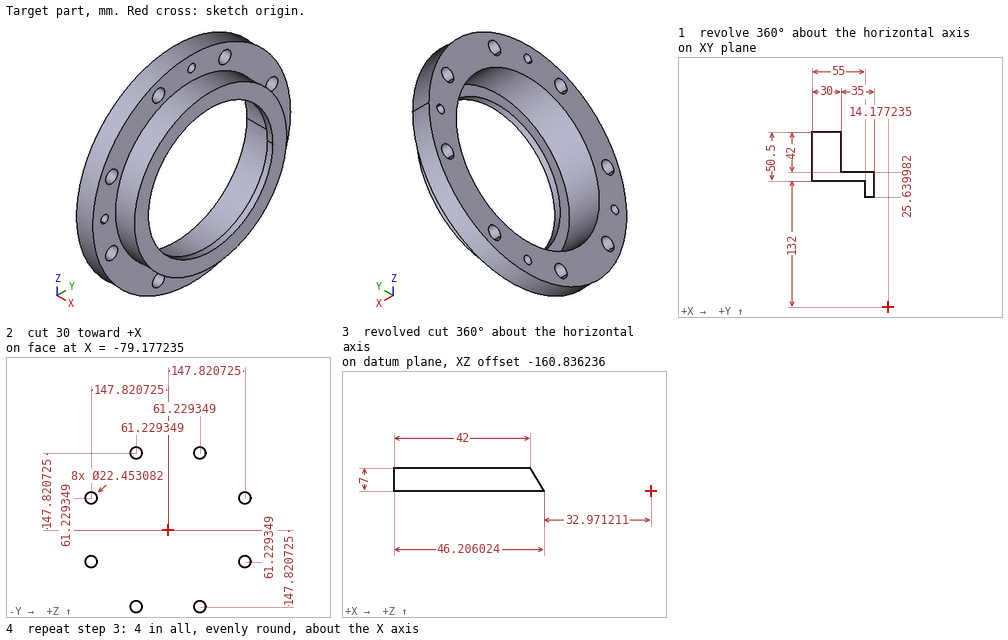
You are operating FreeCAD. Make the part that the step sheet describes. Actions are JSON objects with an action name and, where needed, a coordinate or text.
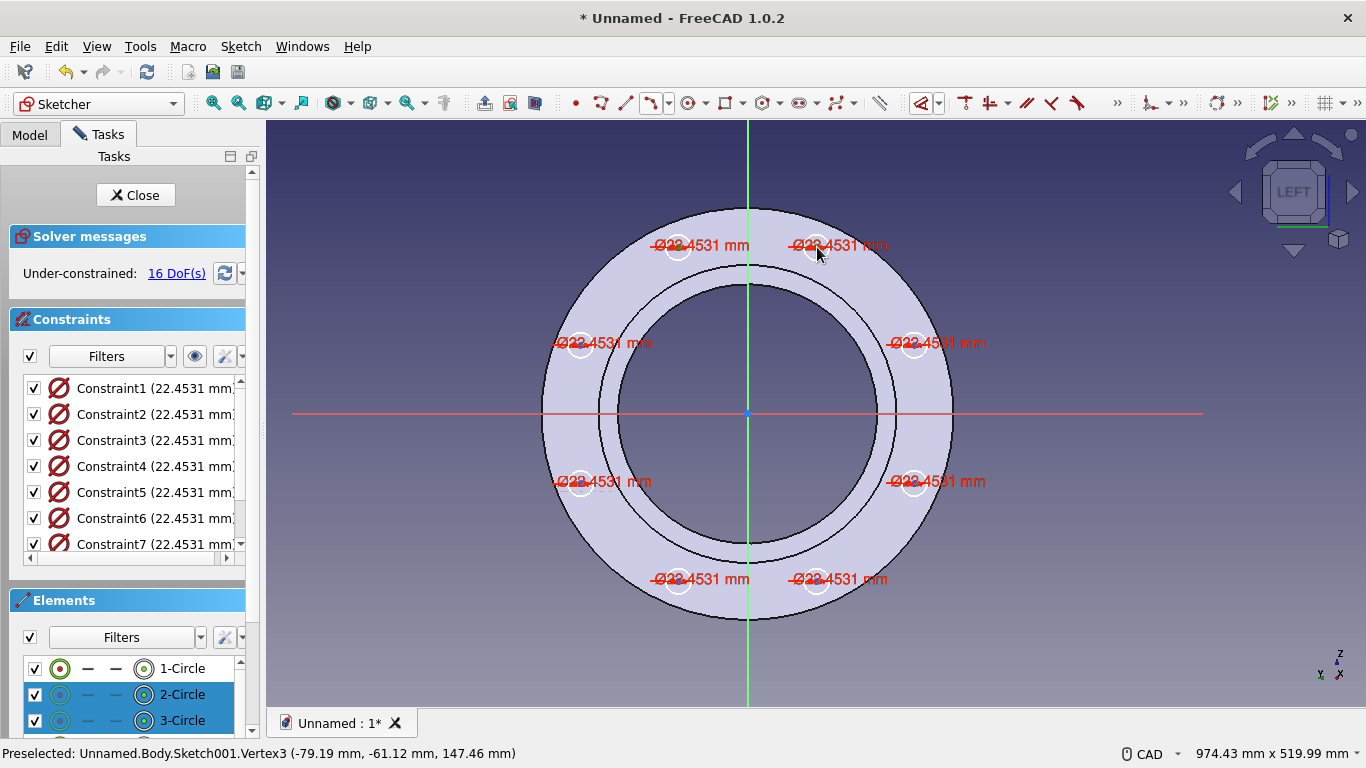
{"action": "left_click", "coordinate": [1008, 104]}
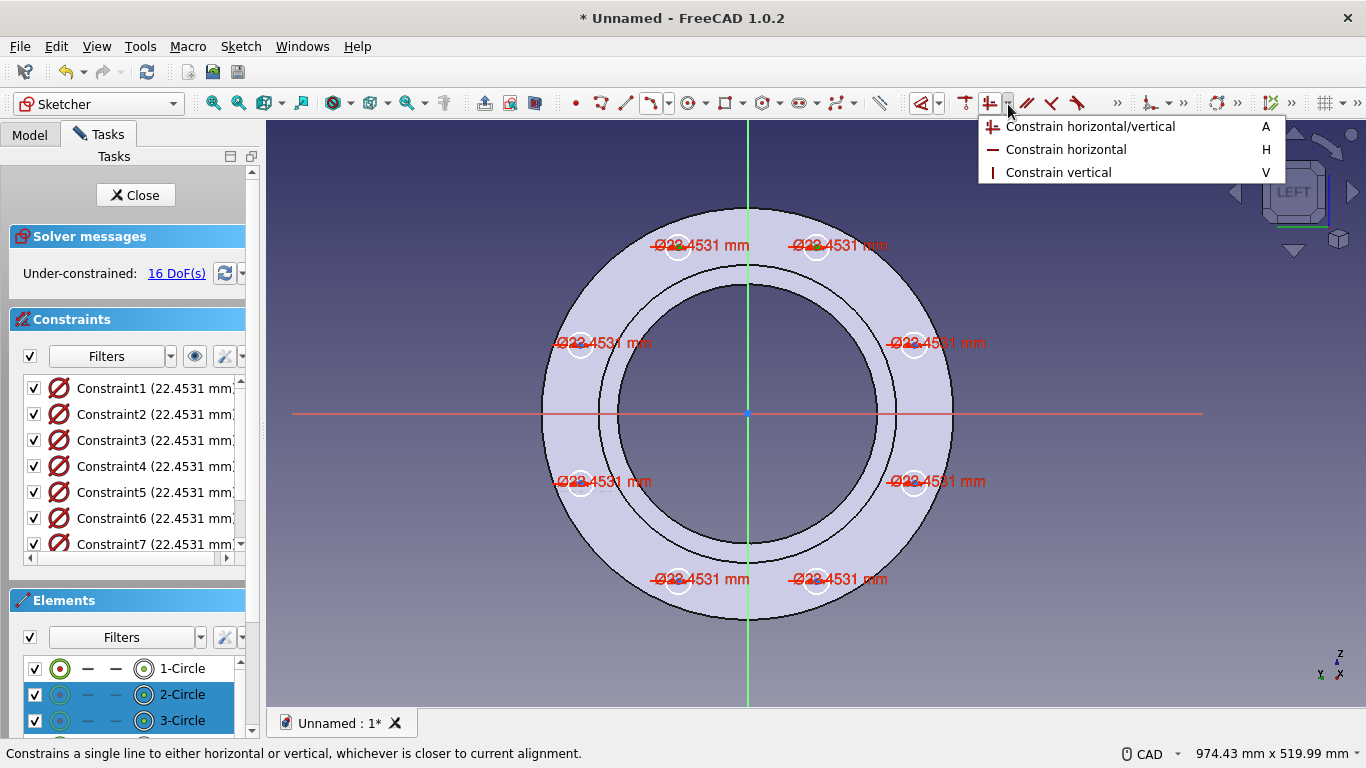
{"action": "left_click", "coordinate": [1132, 150]}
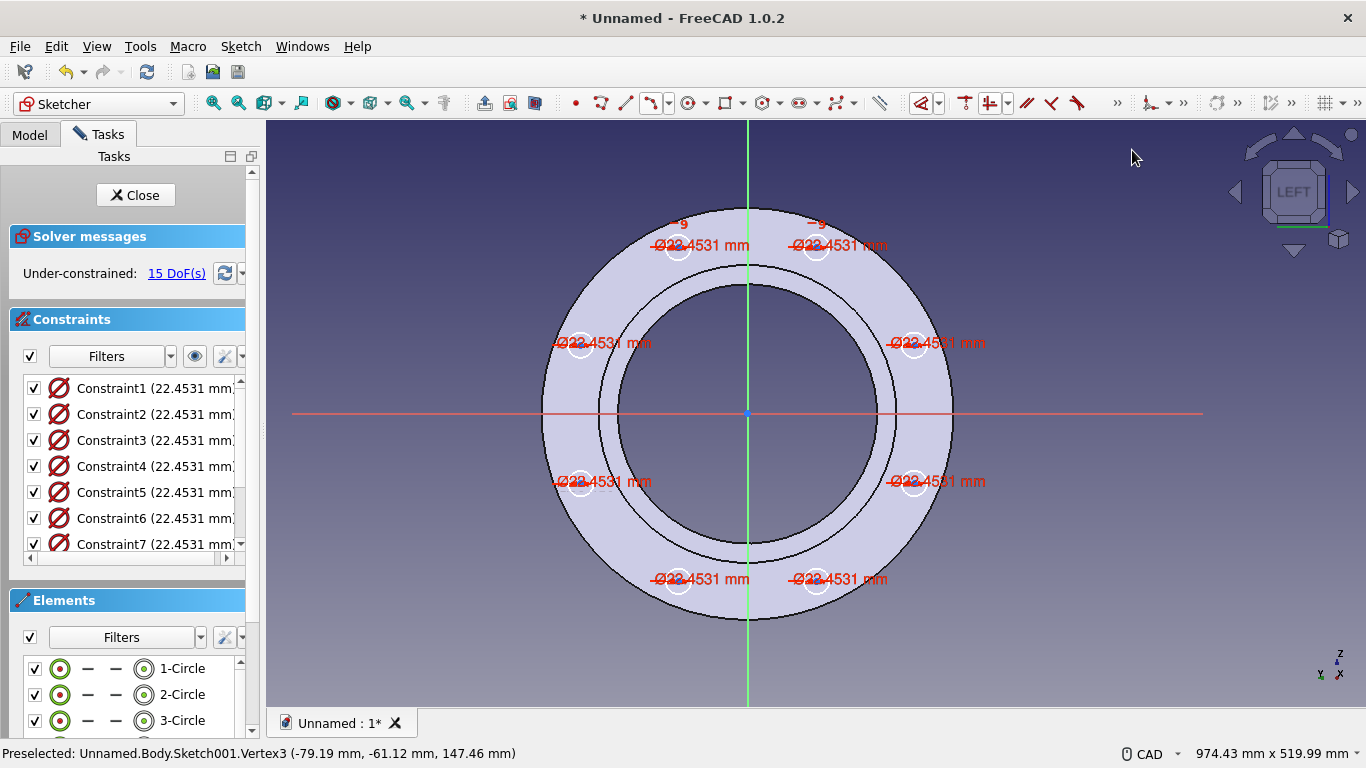
{"action": "left_click", "coordinate": [581, 345]}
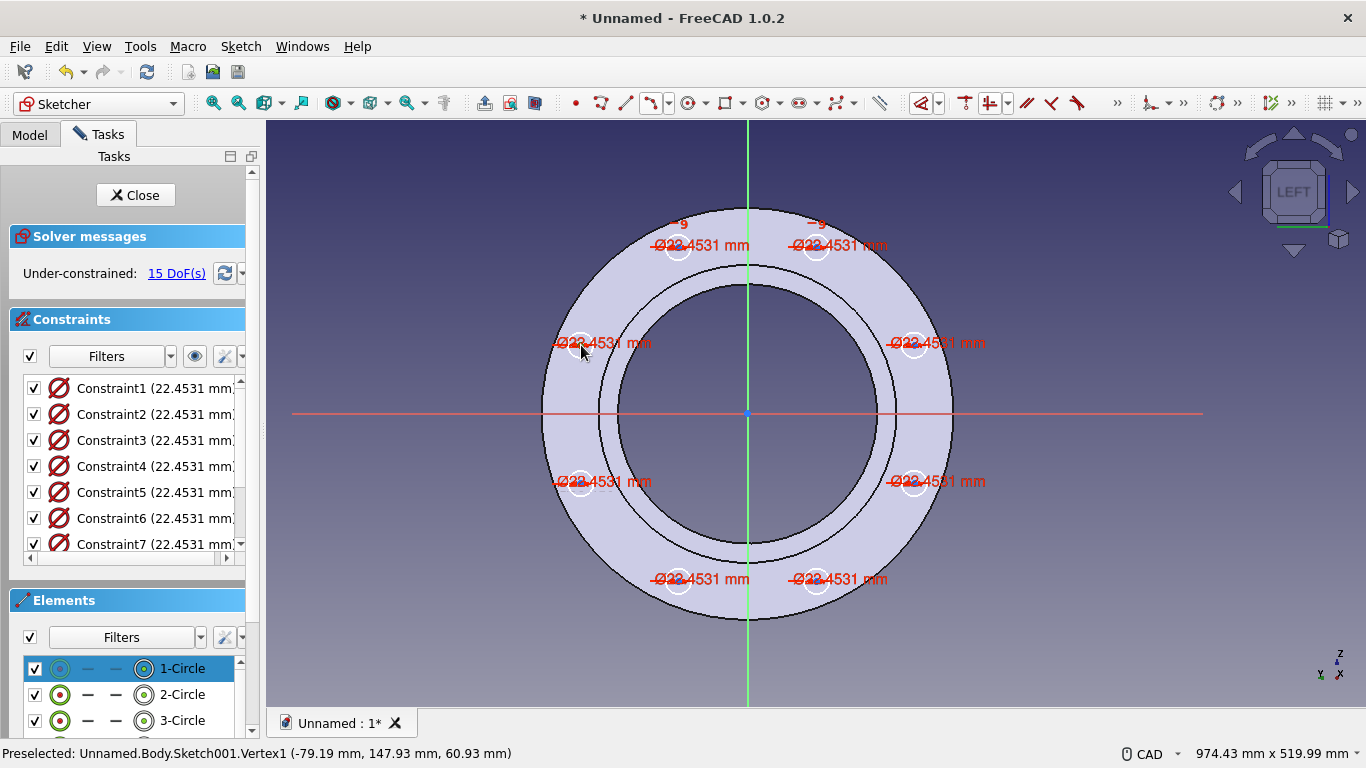
{"action": "left_click", "coordinate": [914, 345]}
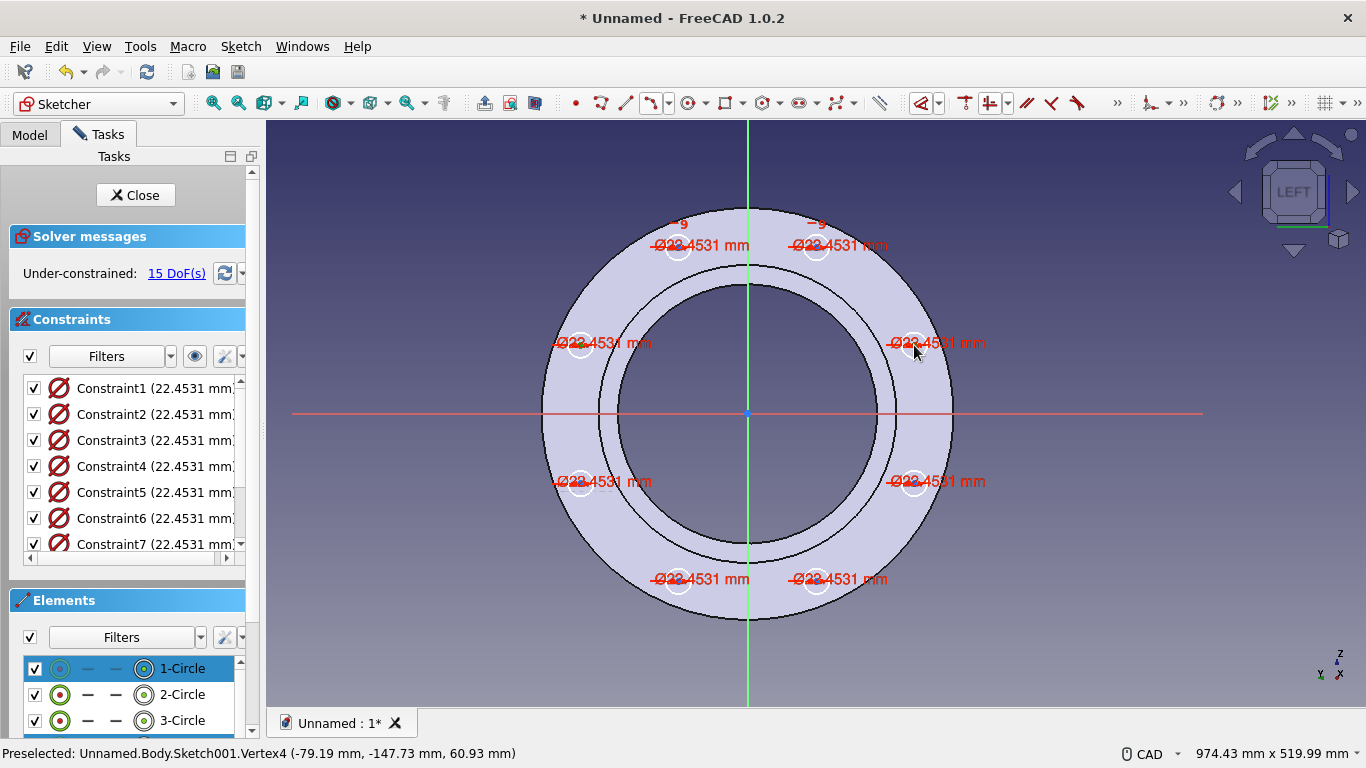
{"action": "key", "text": "h"}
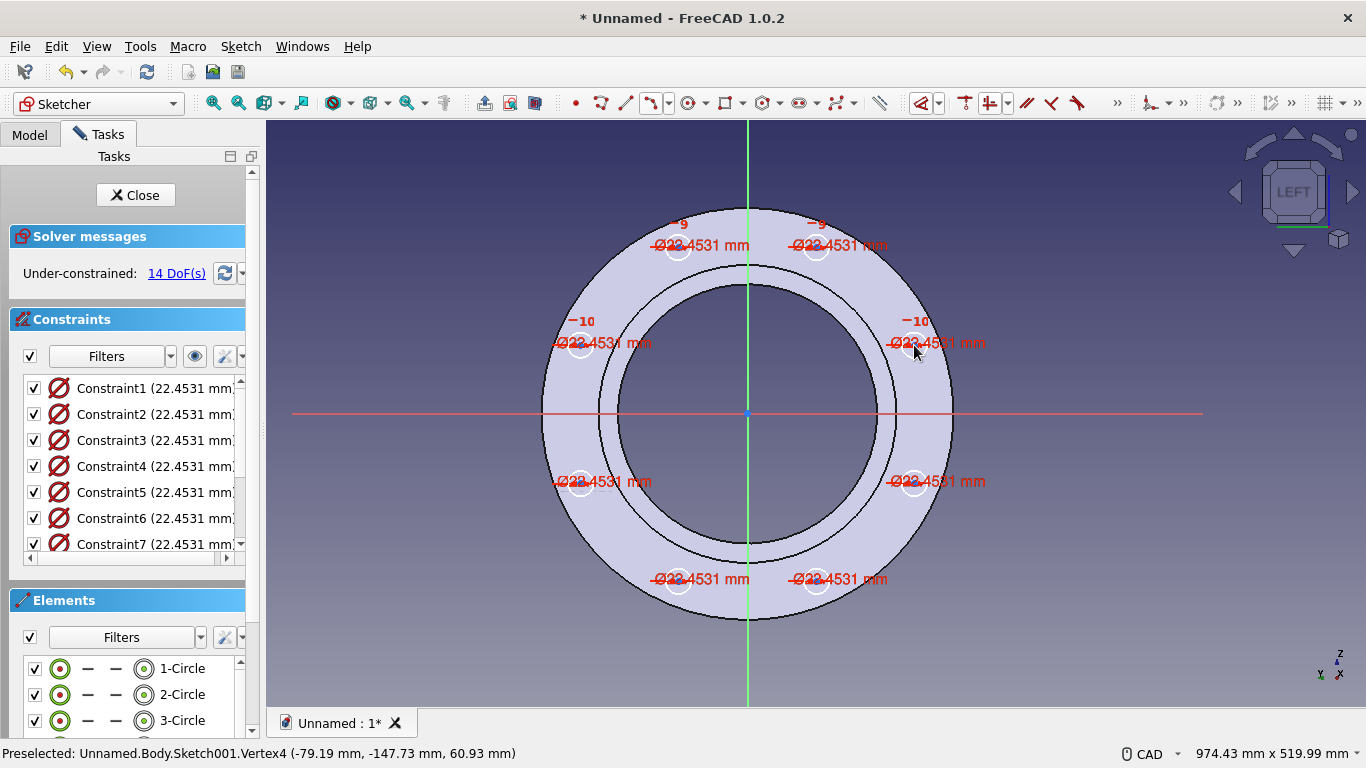
{"action": "left_click", "coordinate": [914, 345]}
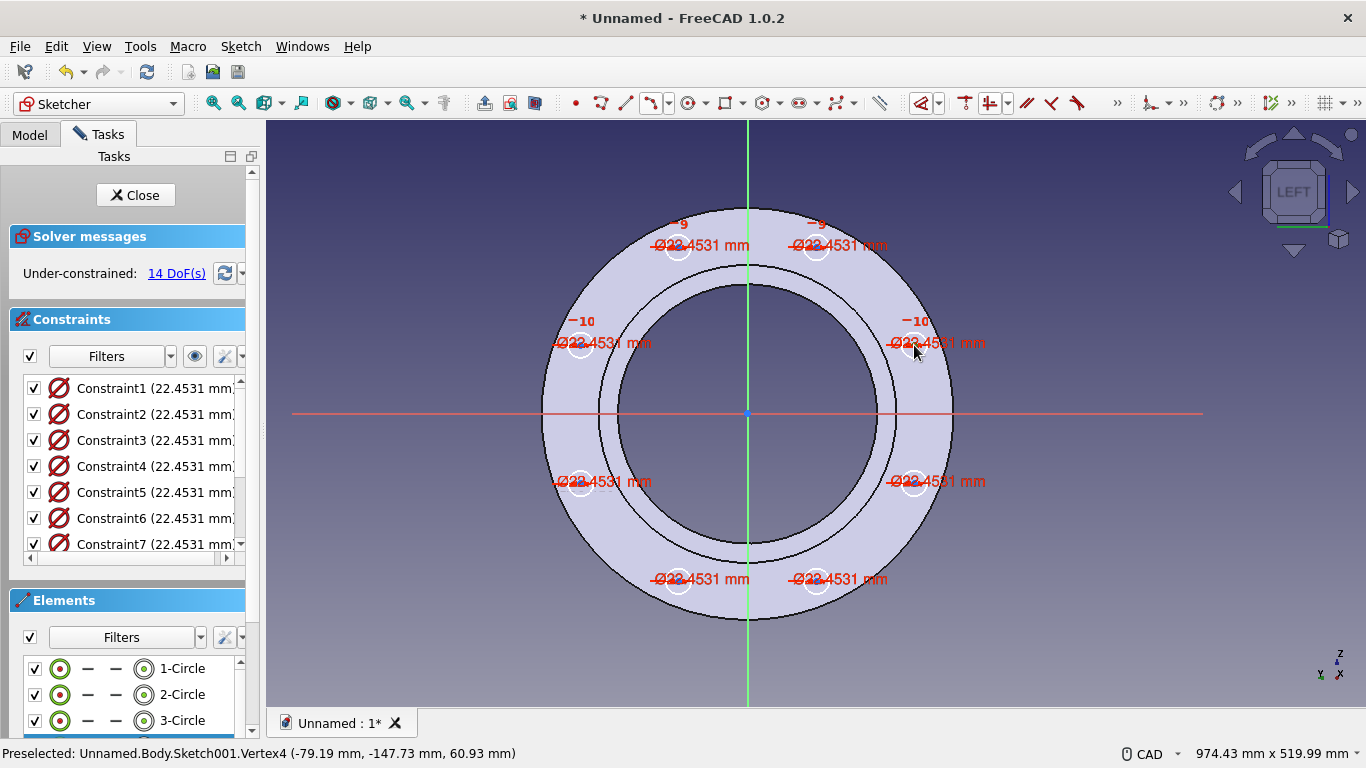
{"action": "left_click", "coordinate": [914, 483]}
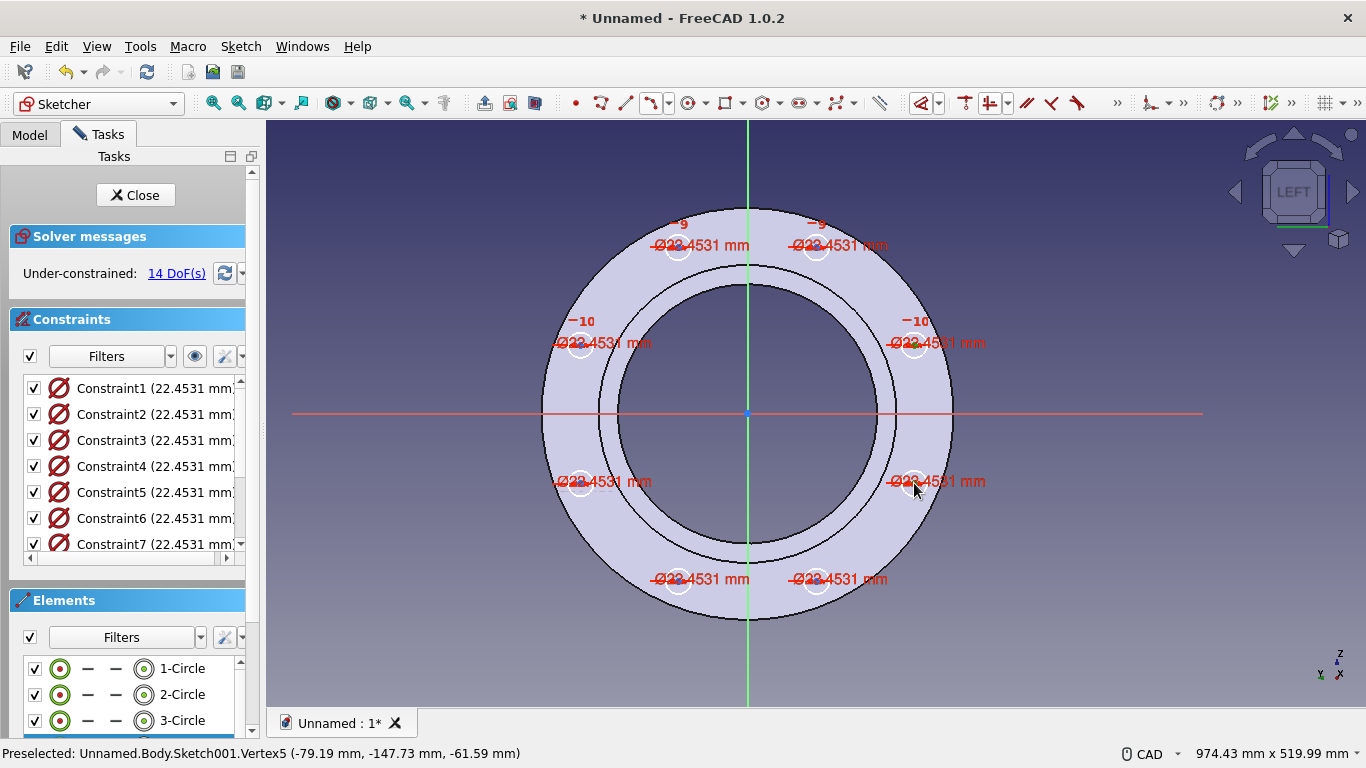
{"action": "left_click", "coordinate": [1008, 104]}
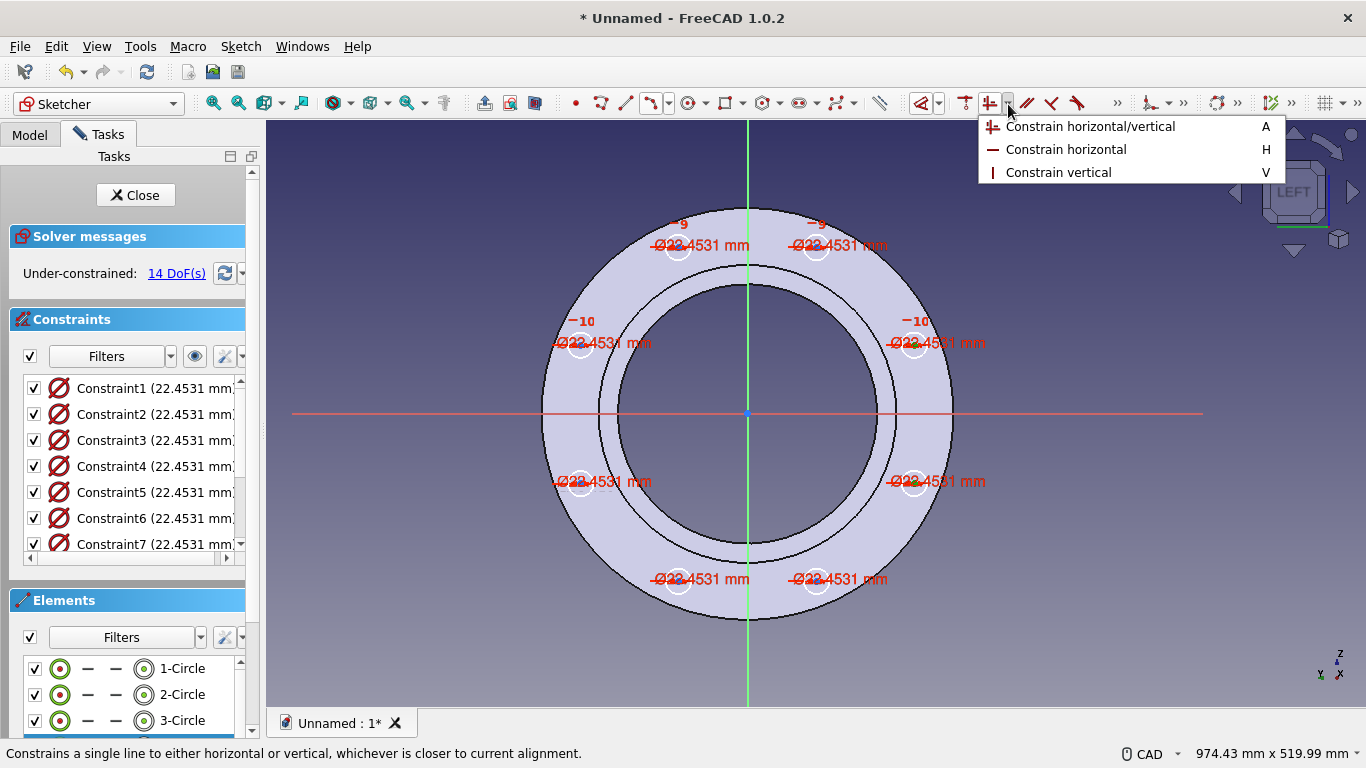
{"action": "left_click", "coordinate": [1132, 172]}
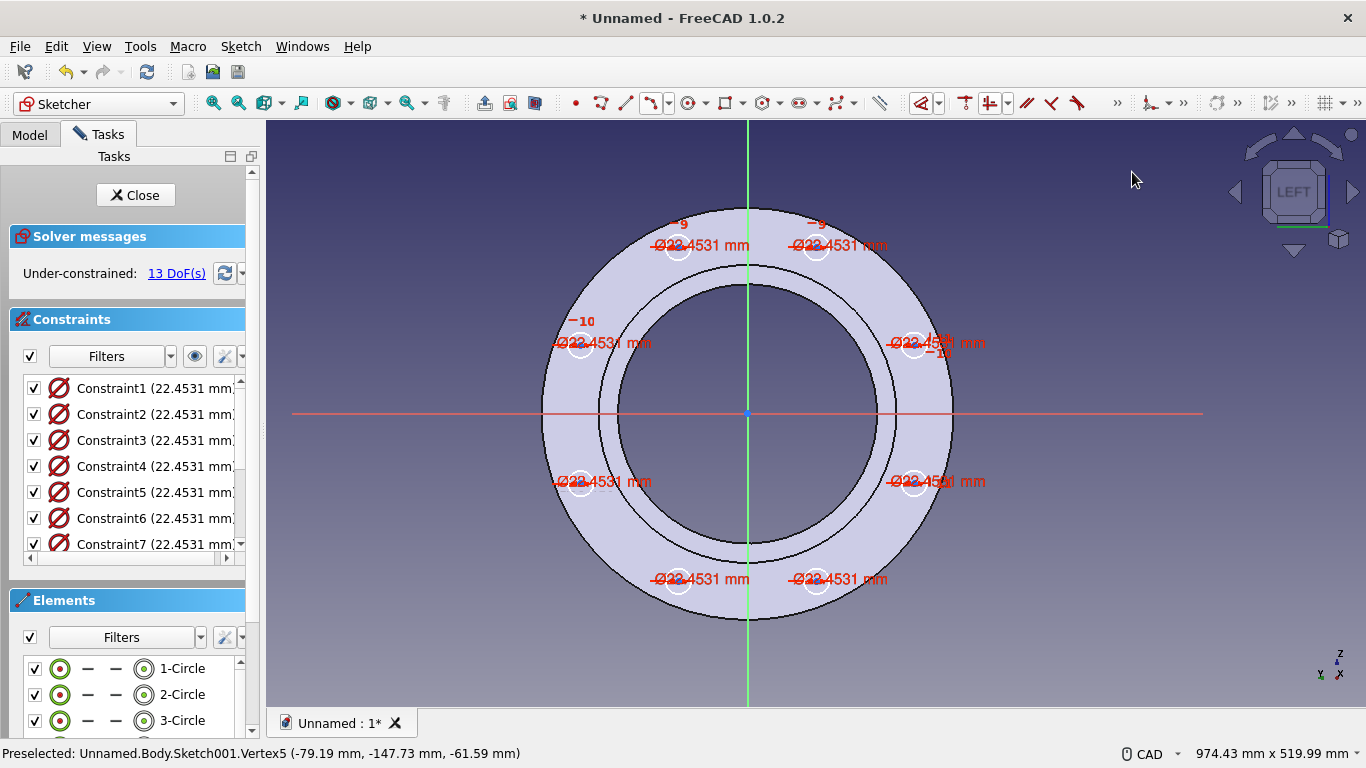
{"action": "left_click", "coordinate": [817, 247]}